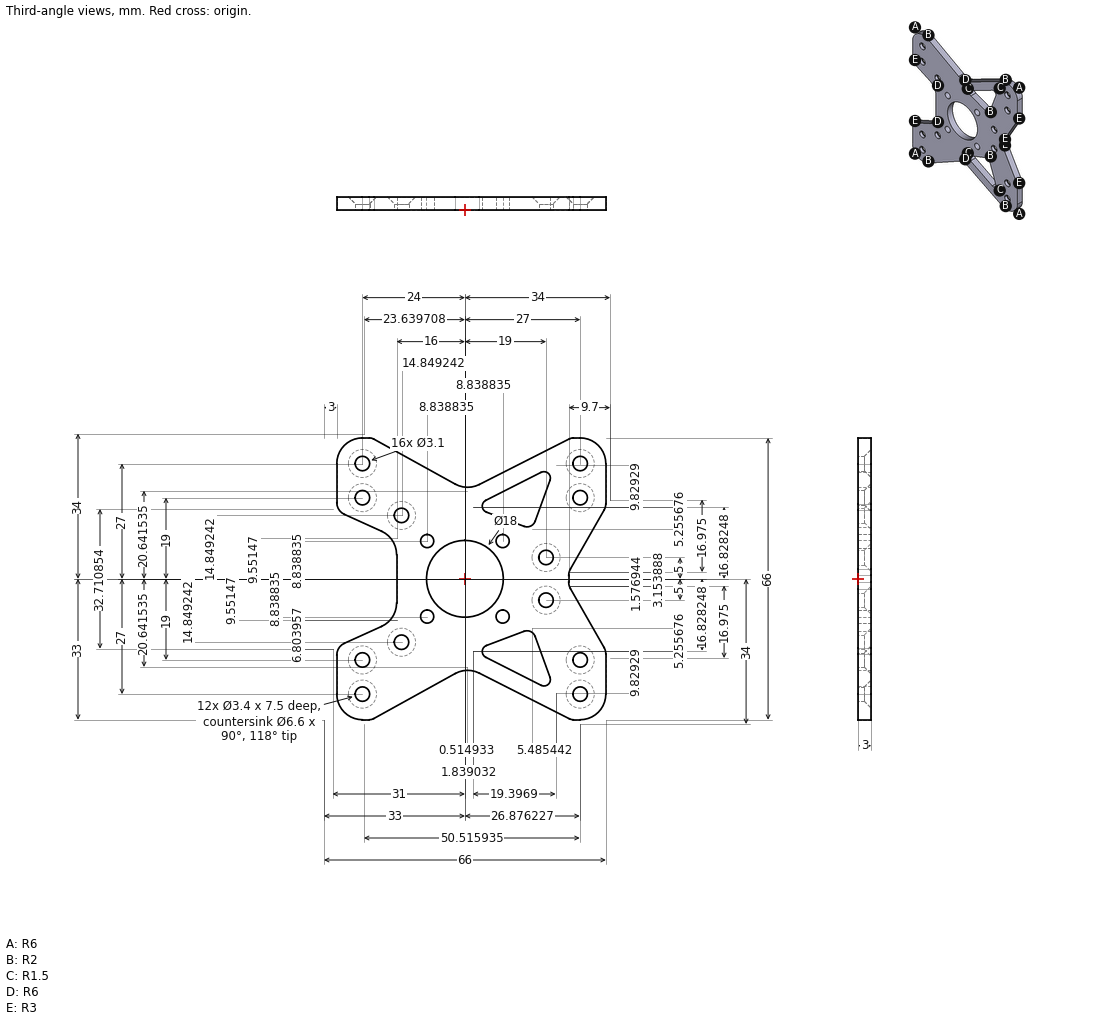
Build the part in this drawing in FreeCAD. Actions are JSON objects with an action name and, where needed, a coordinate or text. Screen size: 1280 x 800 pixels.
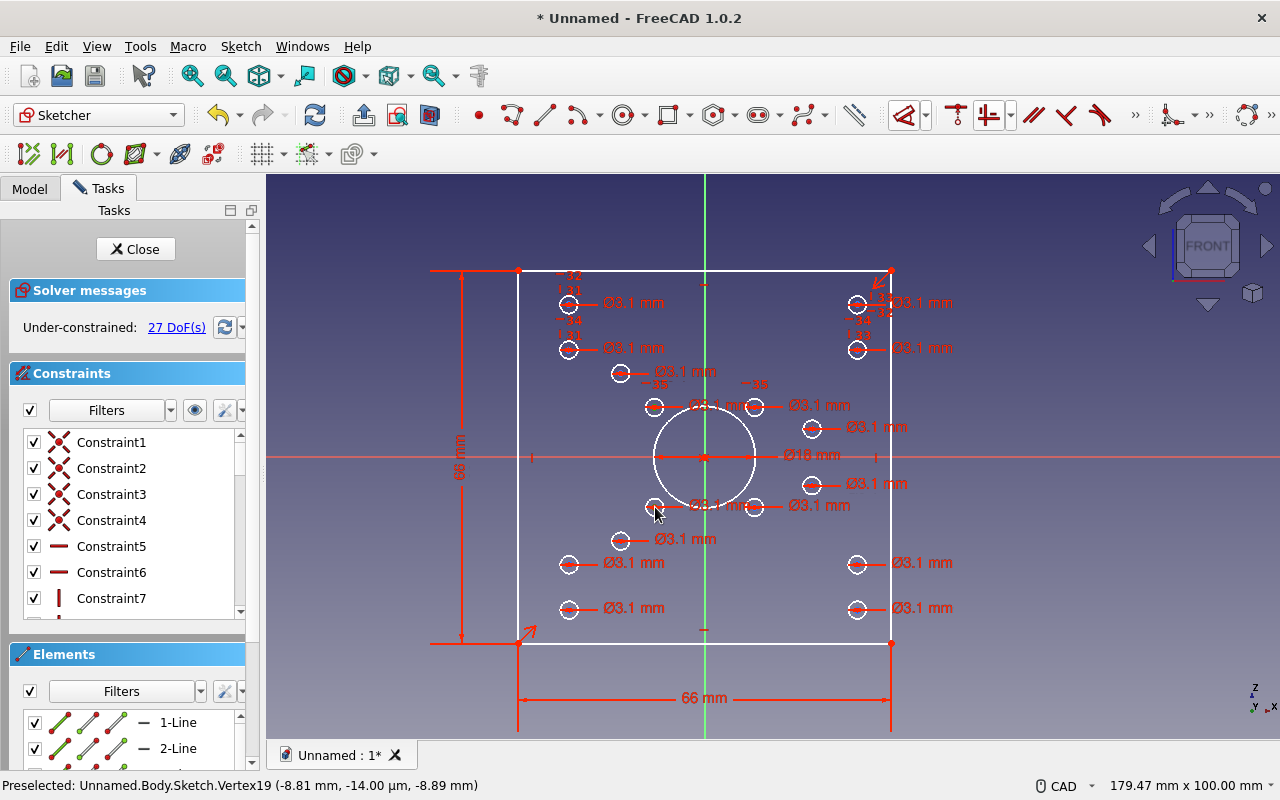
{"action": "key", "text": "v"}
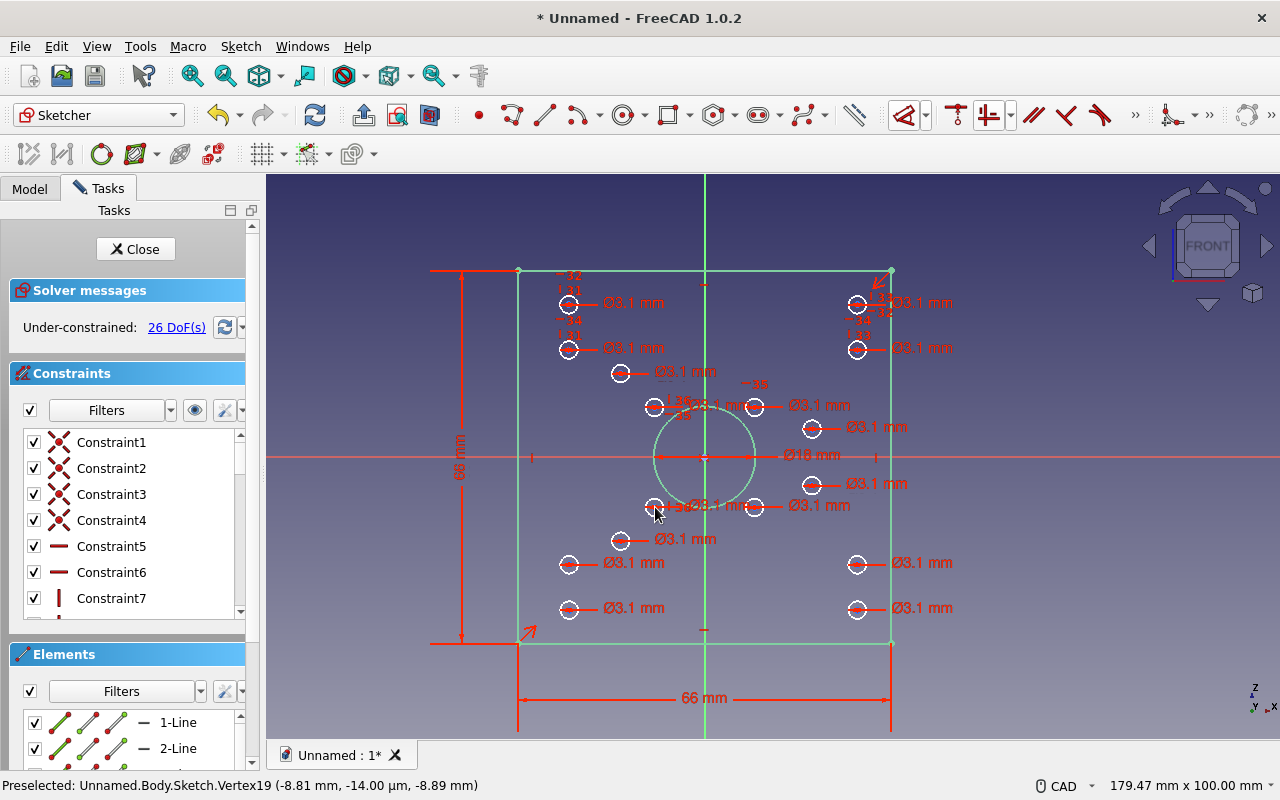
{"action": "left_click", "coordinate": [569, 565]}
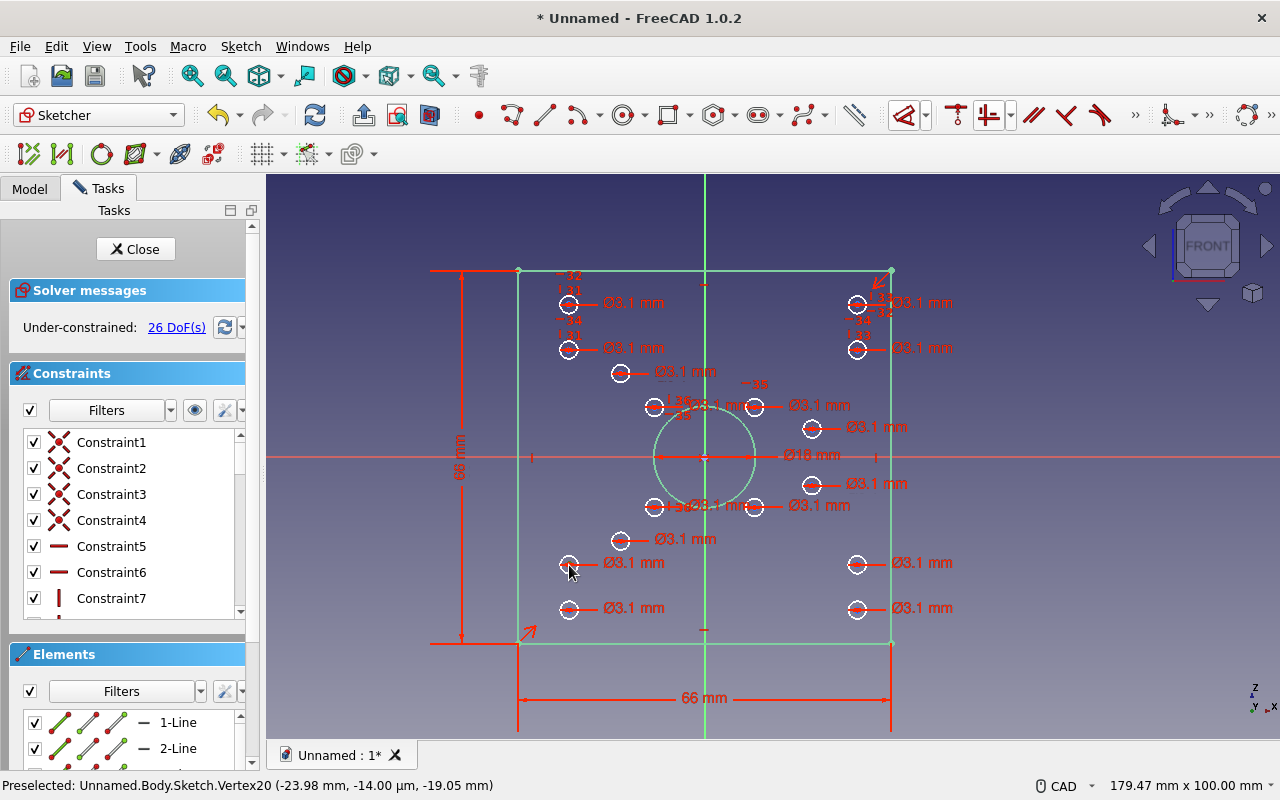
{"action": "left_click", "coordinate": [569, 610]}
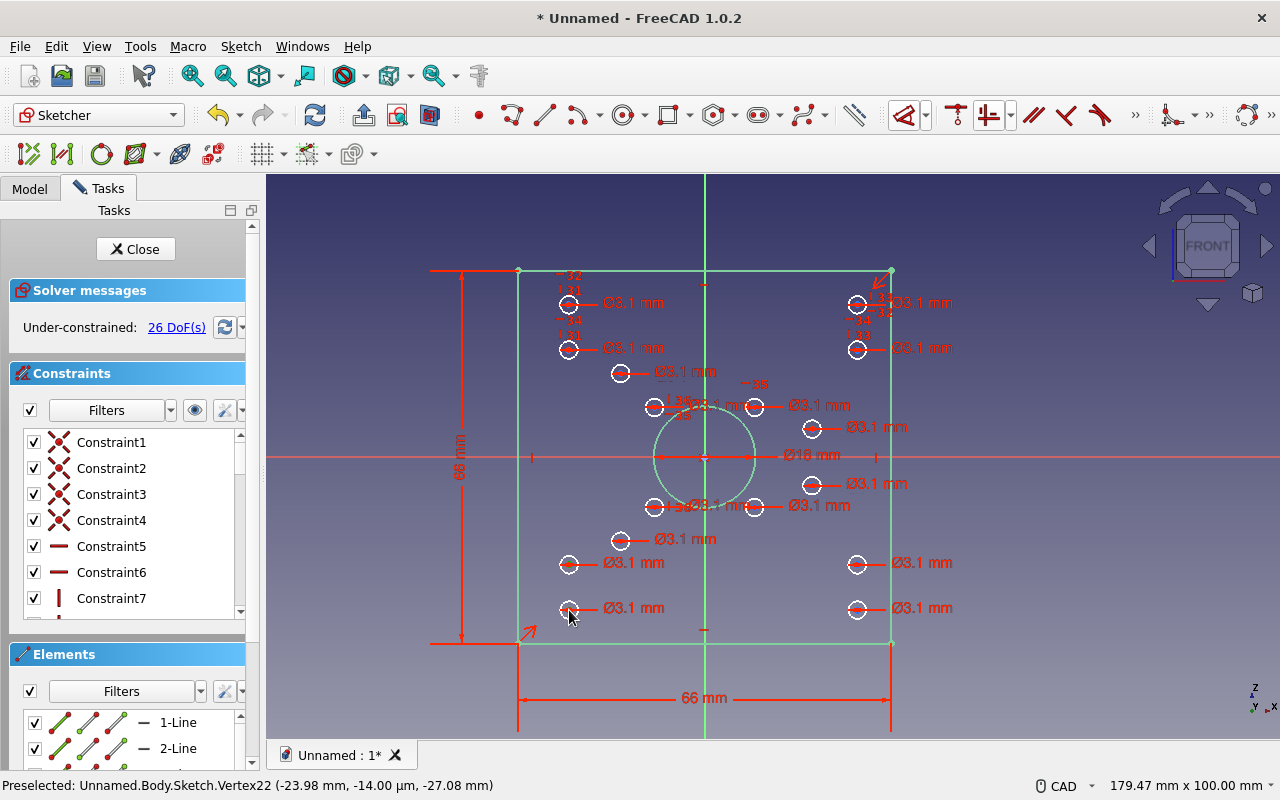
{"action": "key", "text": "v"}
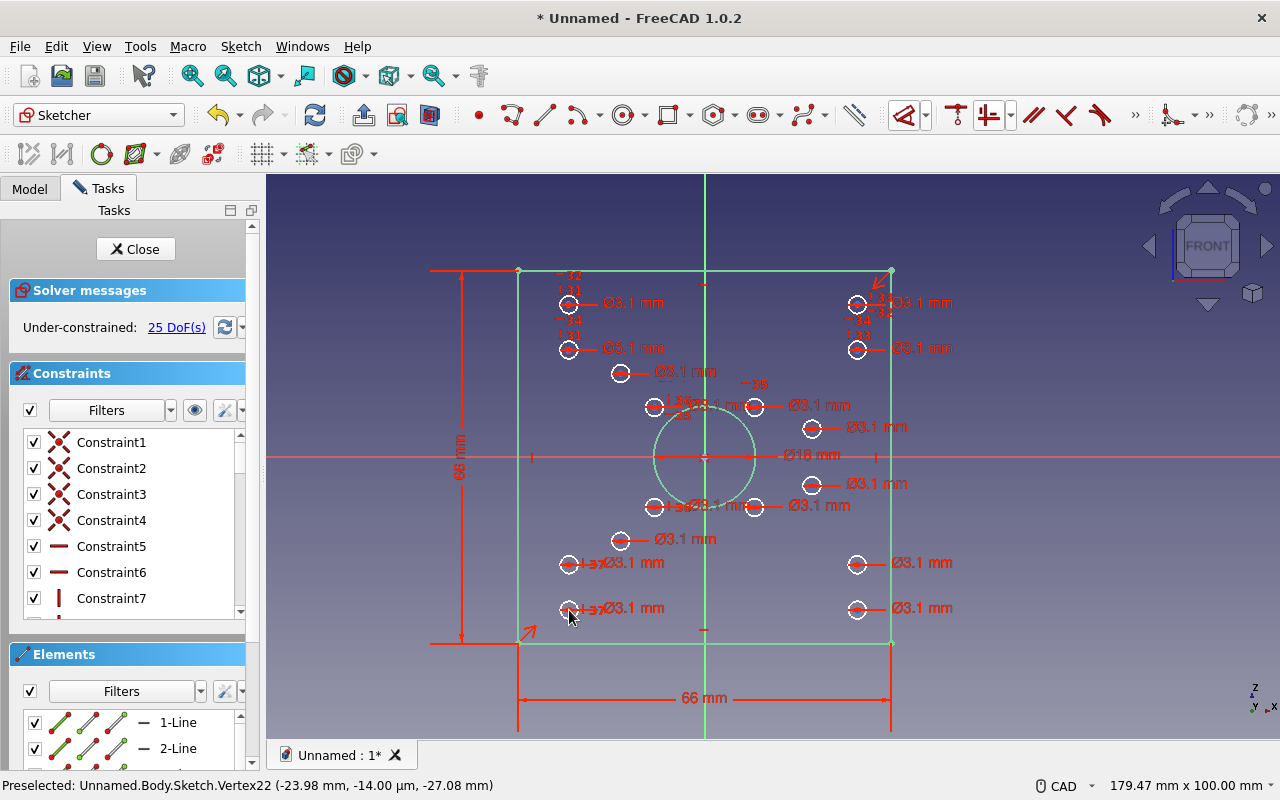
{"action": "left_click", "coordinate": [755, 407]}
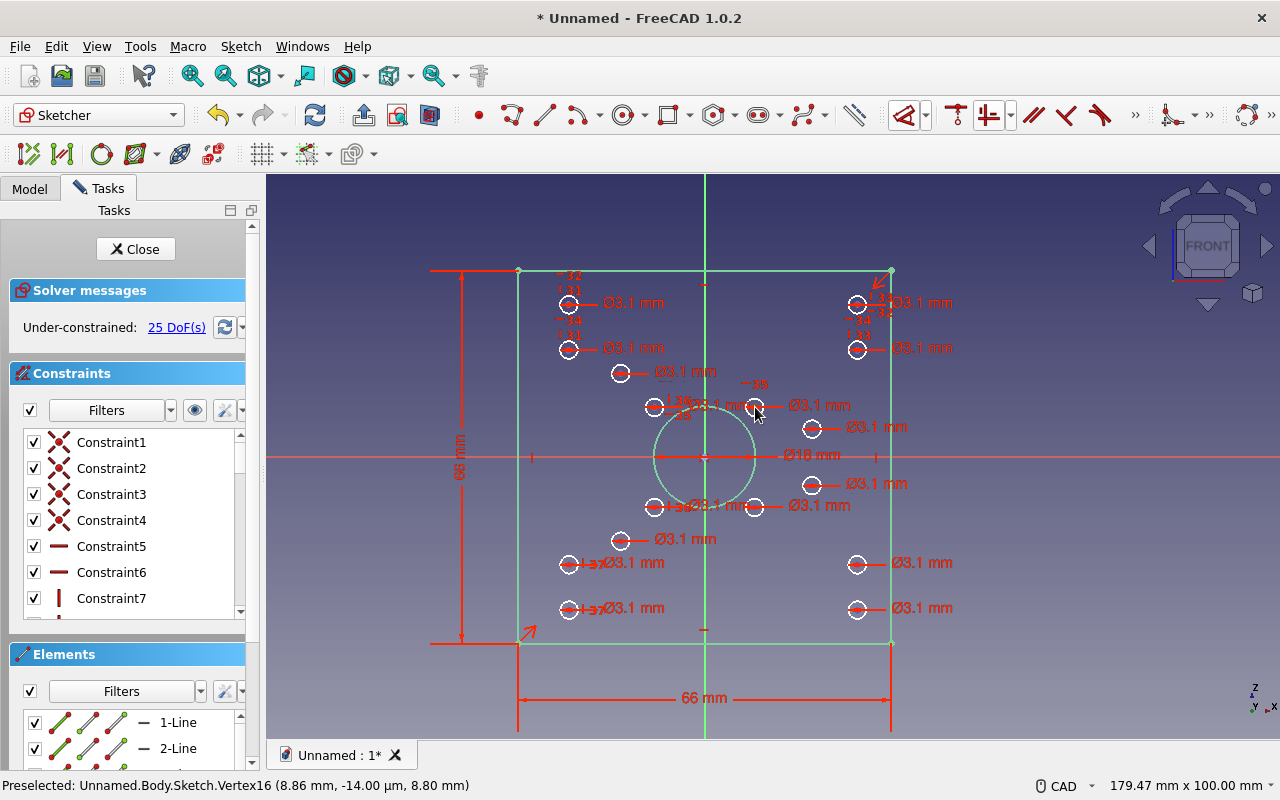
{"action": "left_click", "coordinate": [755, 507]}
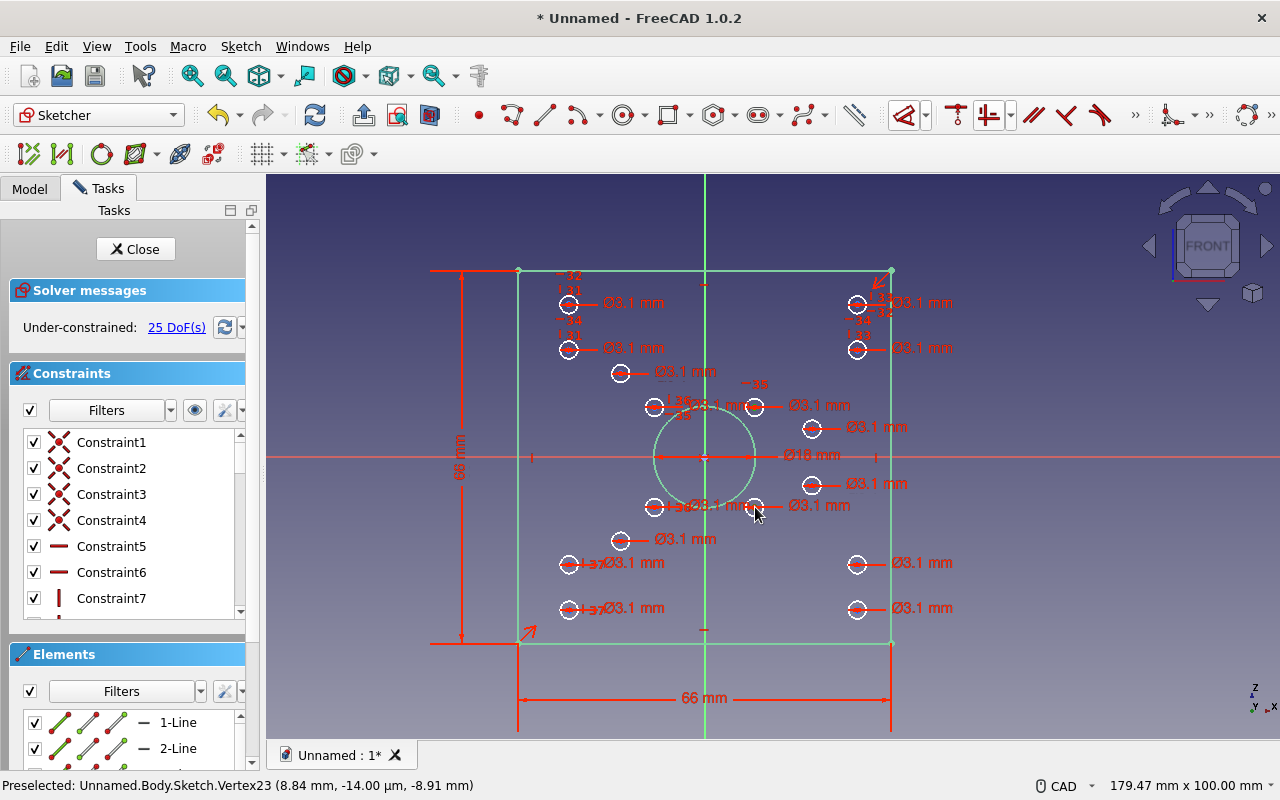
{"action": "key", "text": "v"}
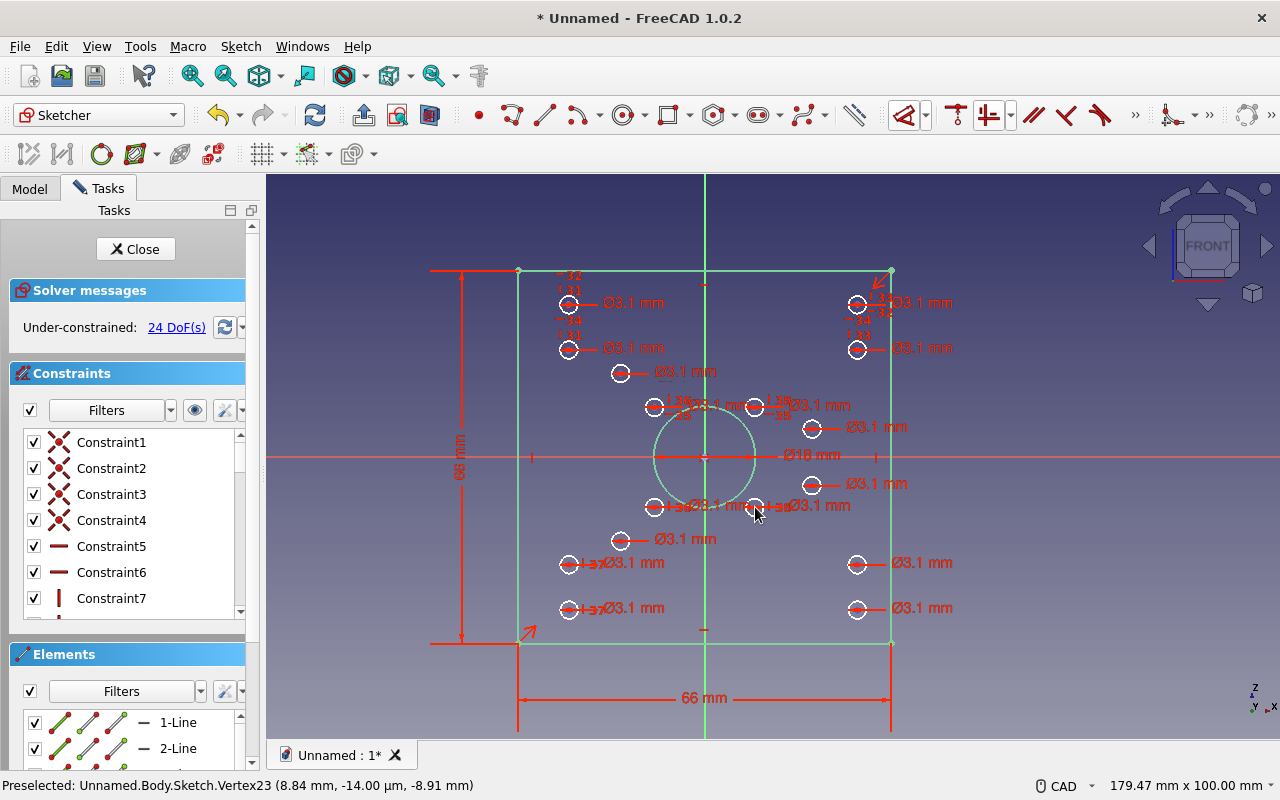
{"action": "left_click", "coordinate": [655, 507]}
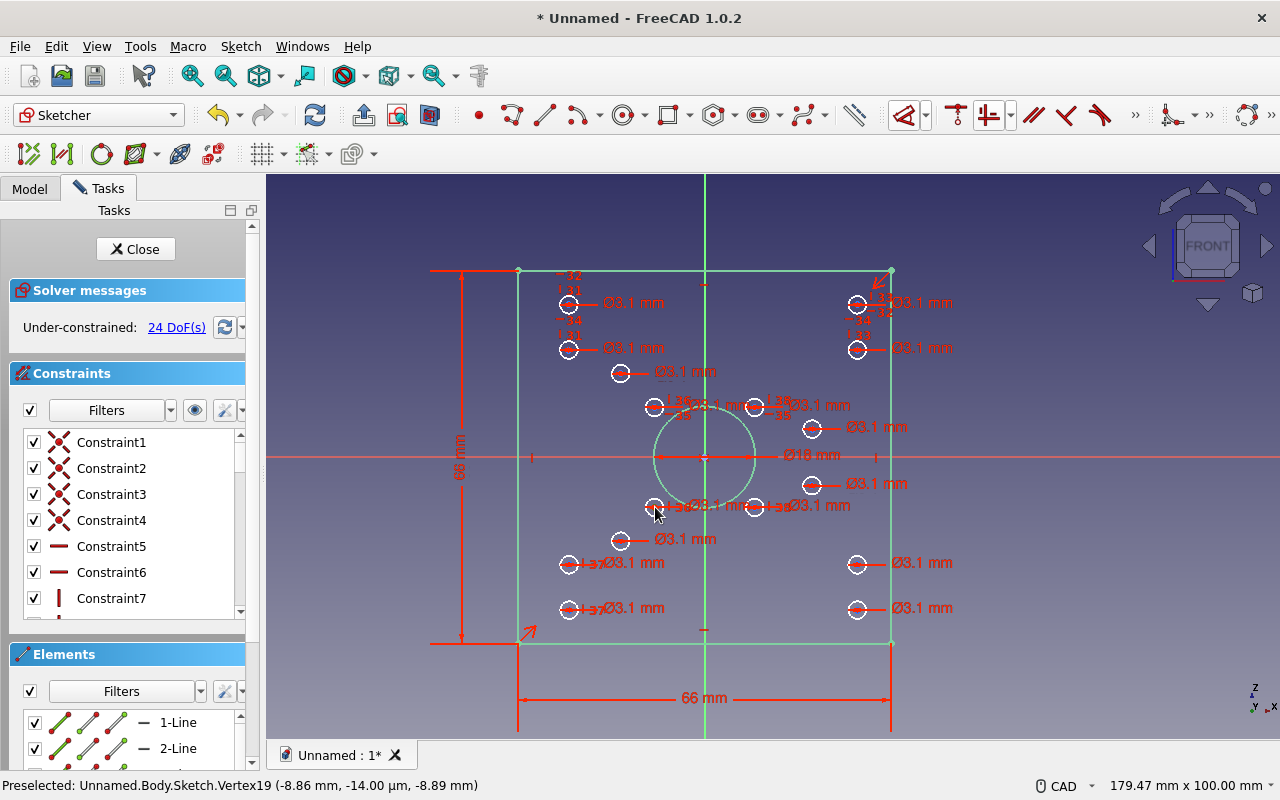
{"action": "left_click", "coordinate": [755, 507]}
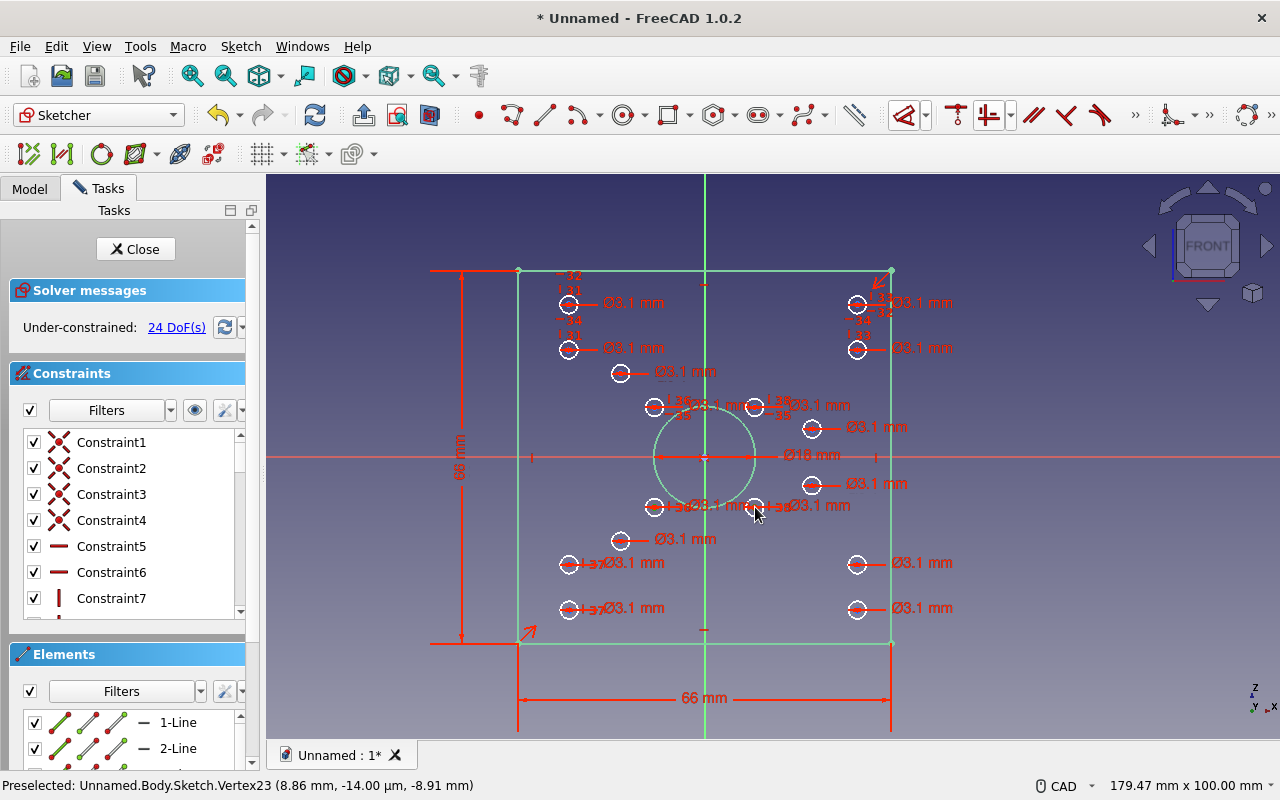
{"action": "key", "text": "h"}